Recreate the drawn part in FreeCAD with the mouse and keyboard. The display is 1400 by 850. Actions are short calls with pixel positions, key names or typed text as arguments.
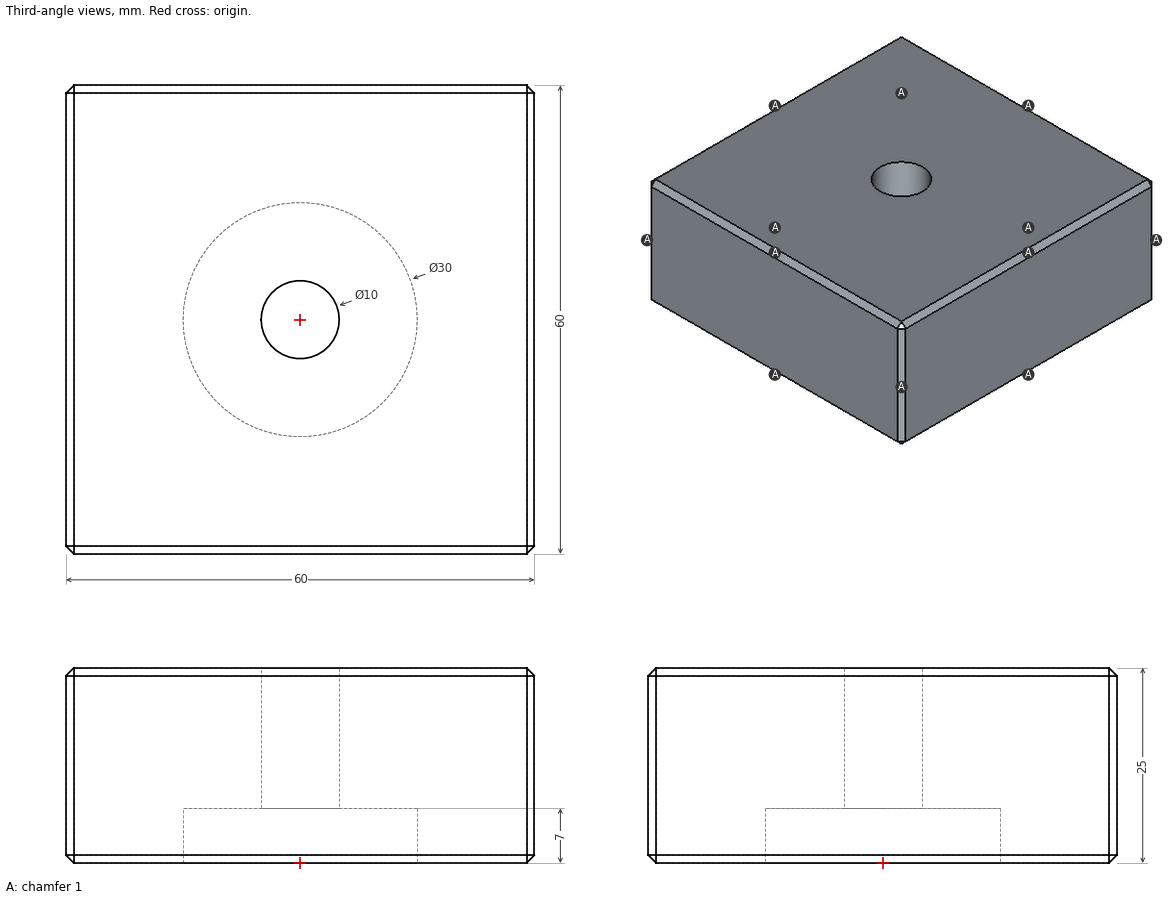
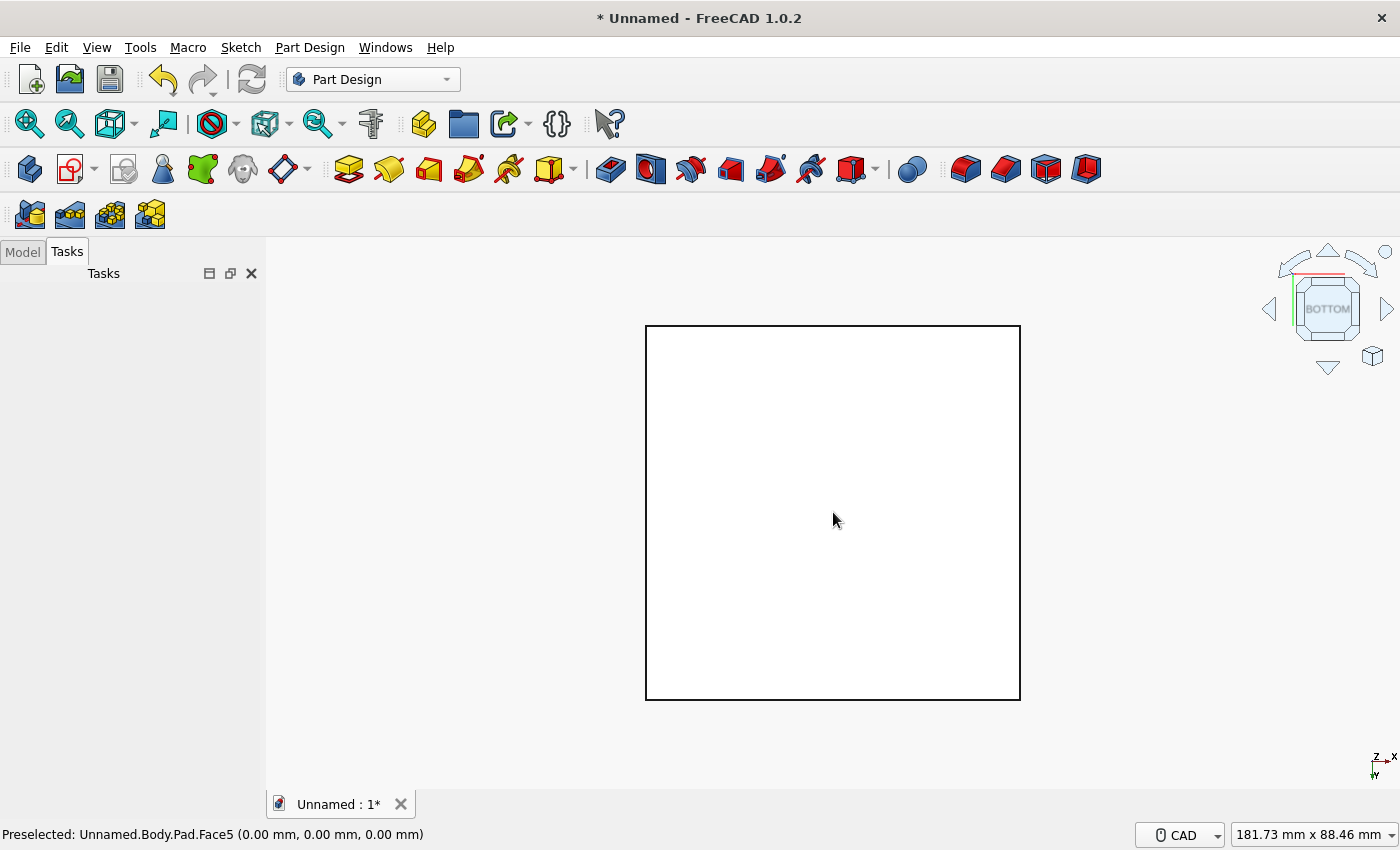
key(4)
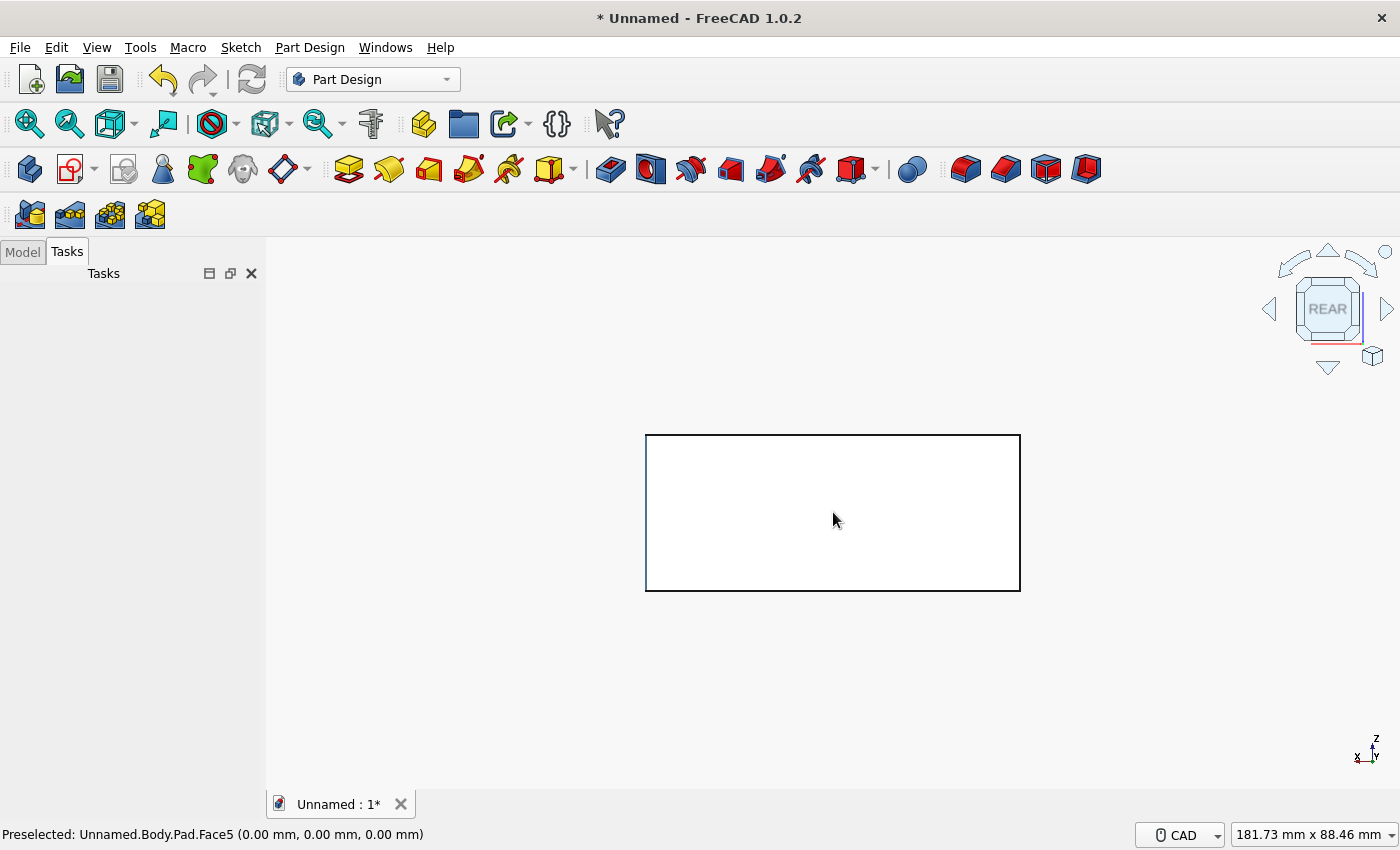
click(30, 124)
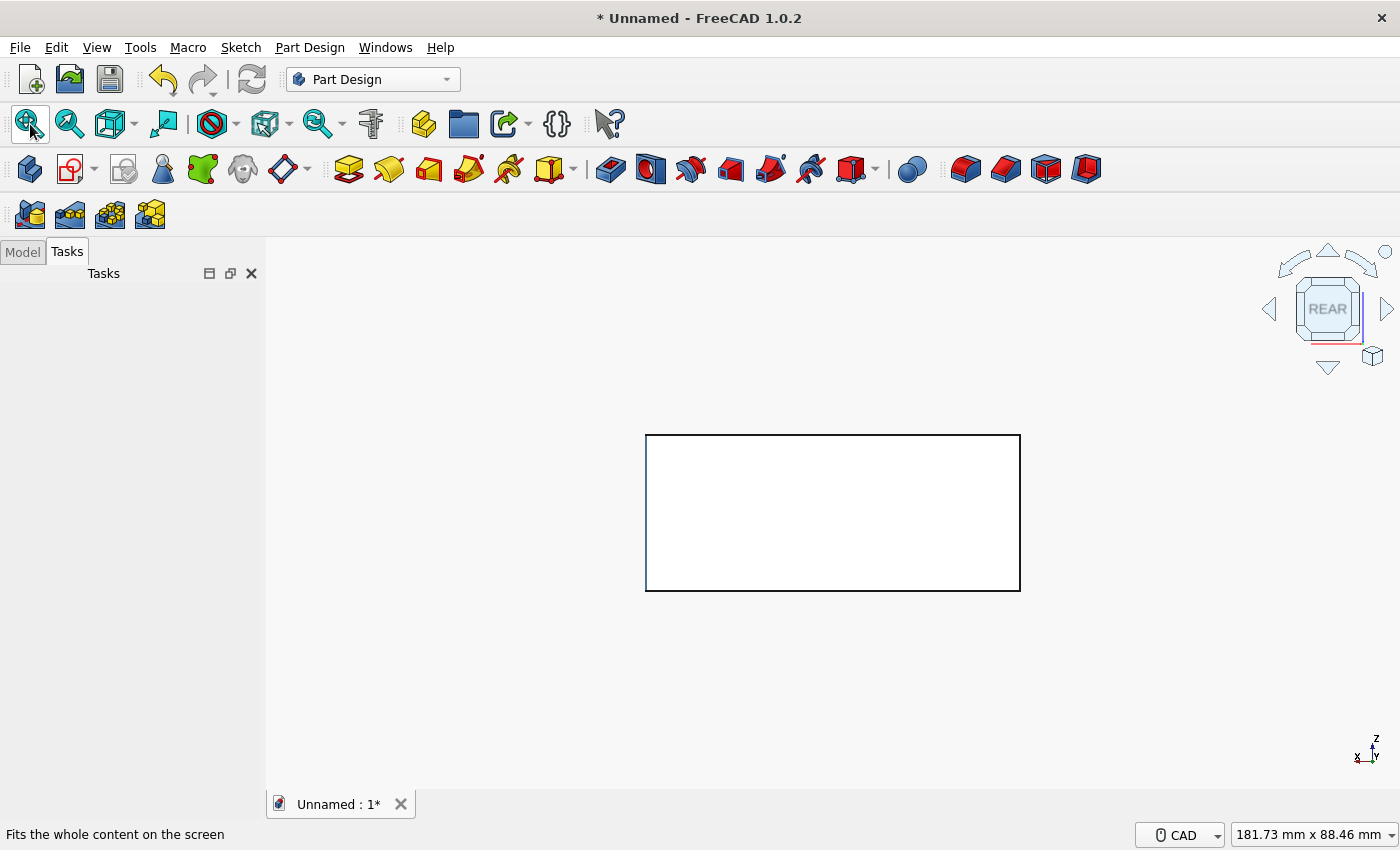
click(1020, 512, ctrl)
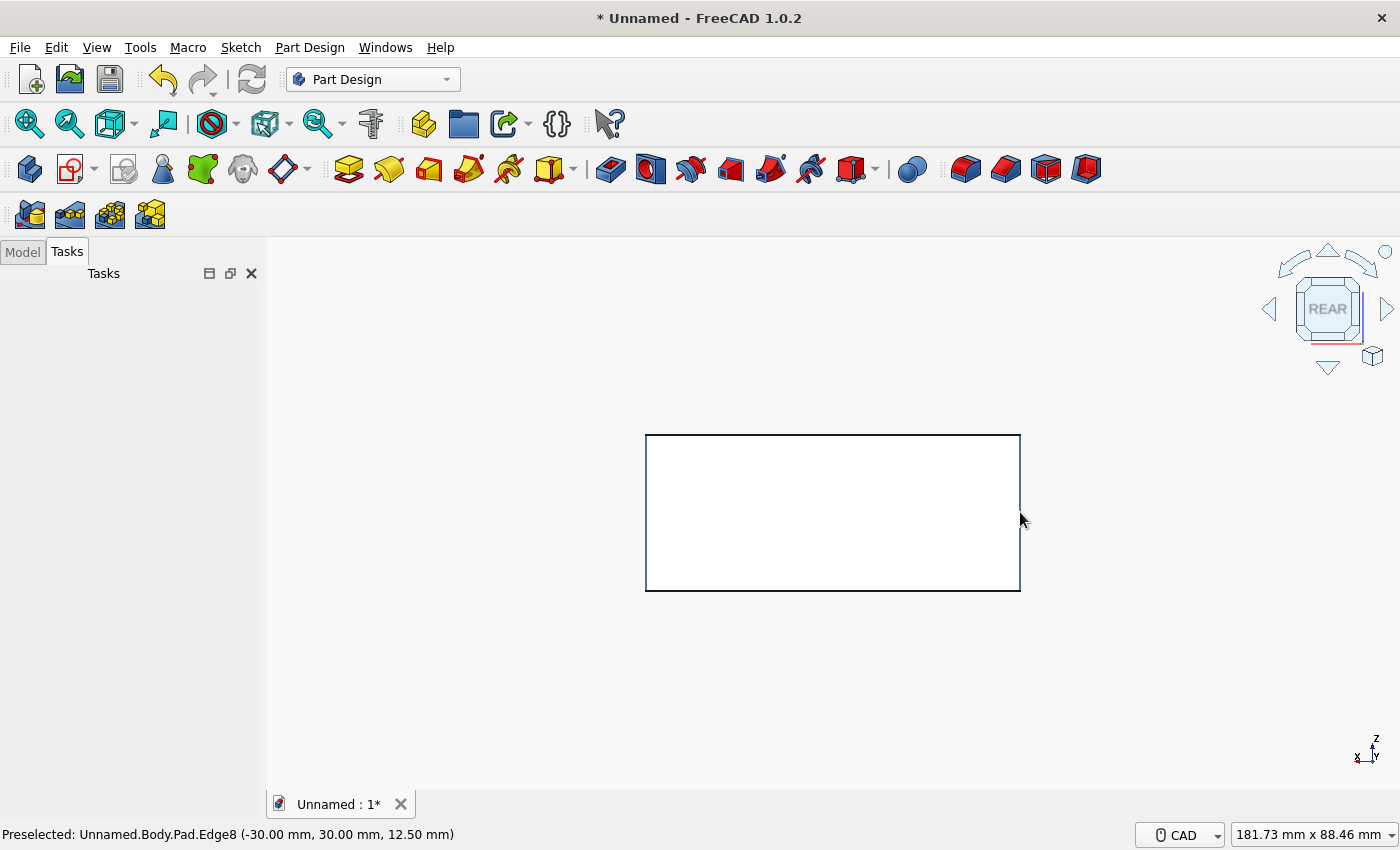
click(1006, 170)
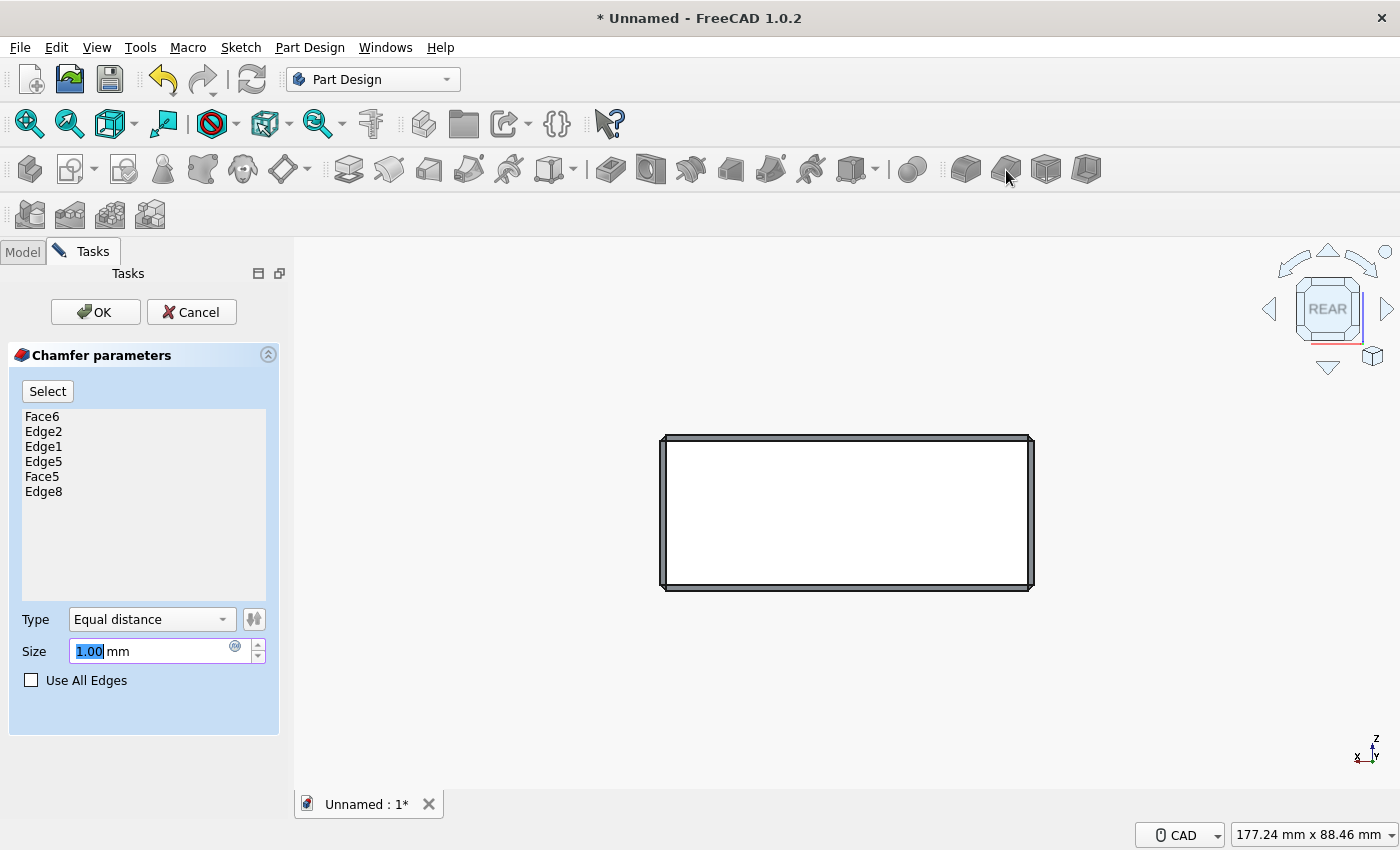
text(1)
key(Tab)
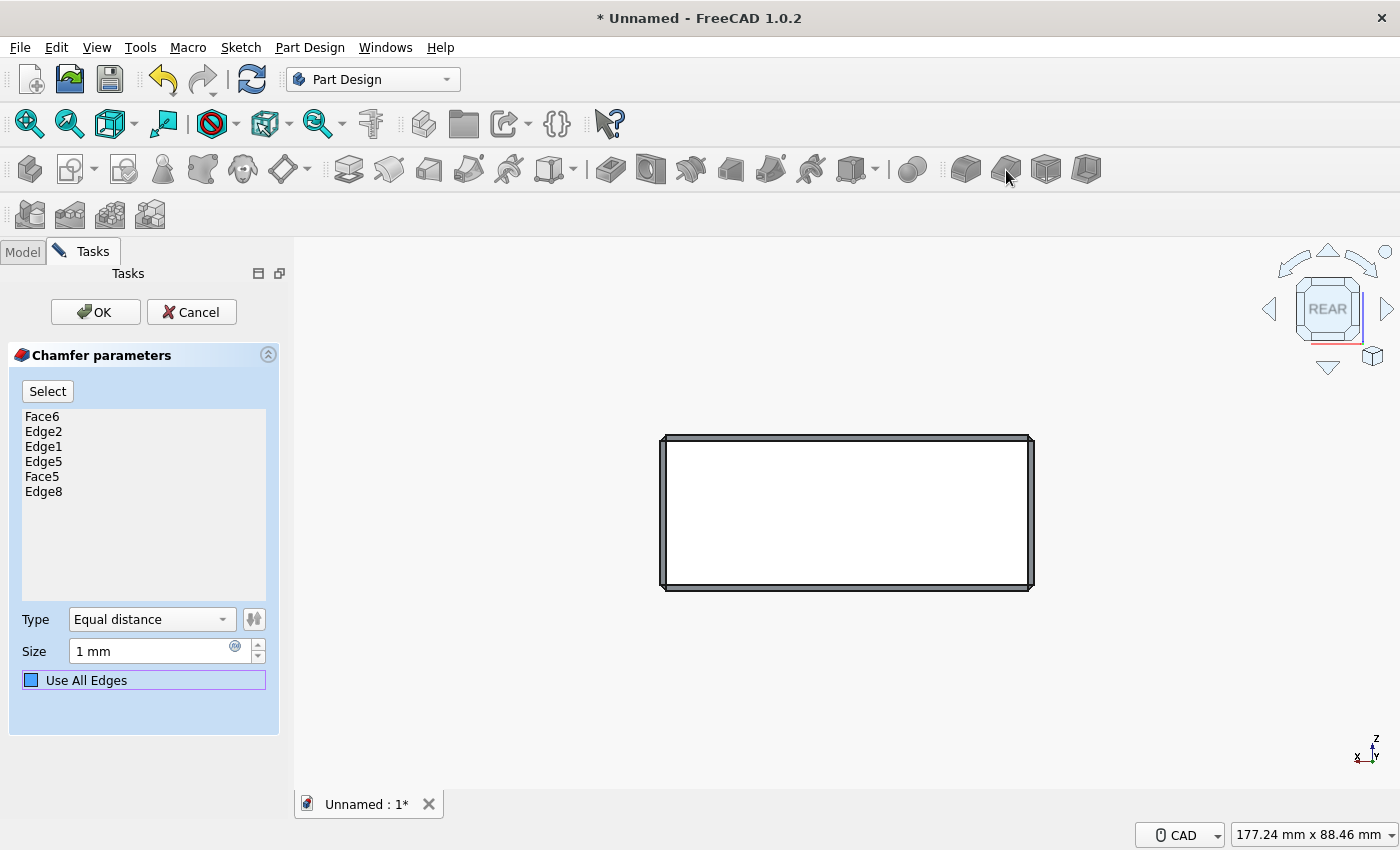
click(96, 312)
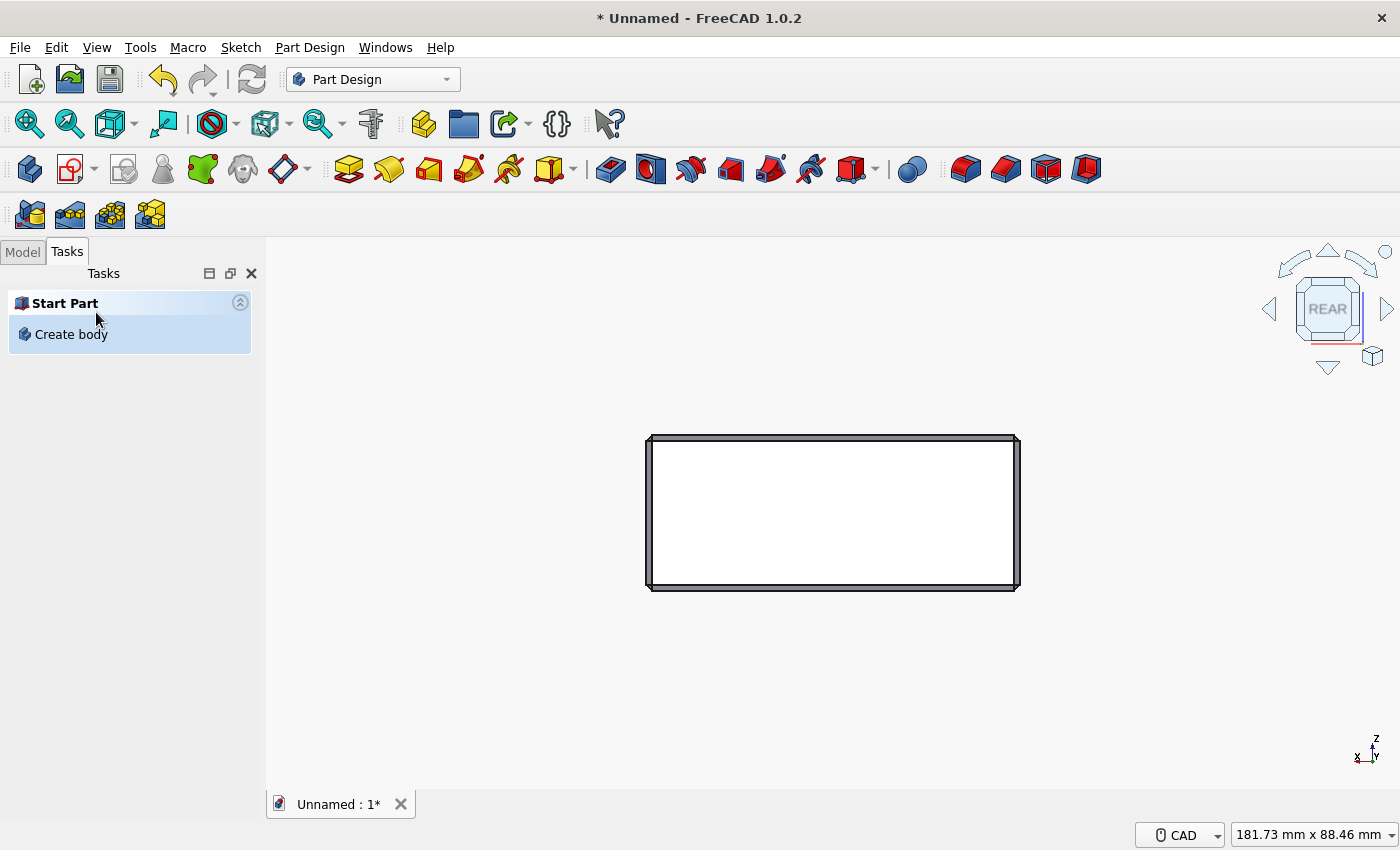
key(v)
key(f)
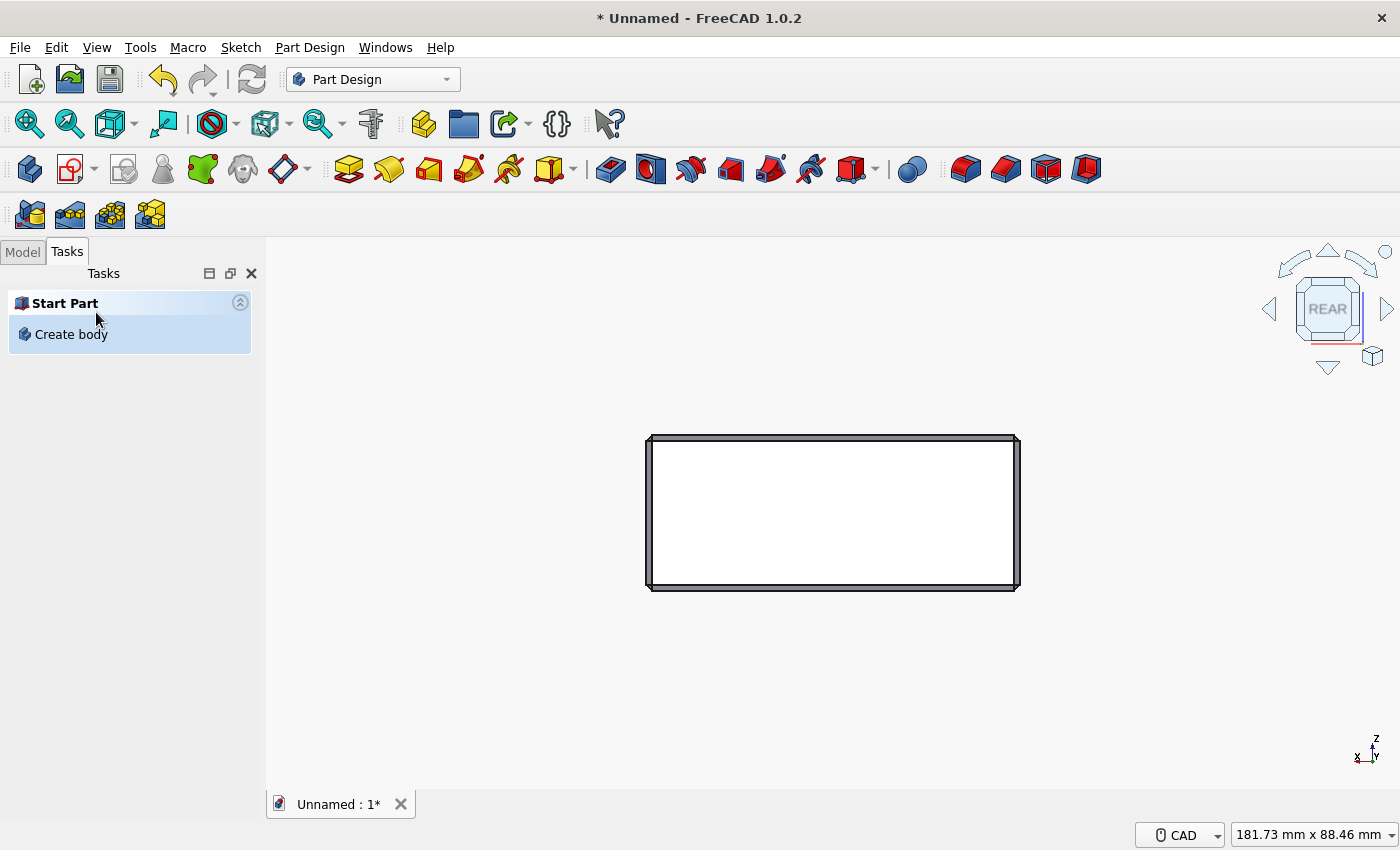
key(5)